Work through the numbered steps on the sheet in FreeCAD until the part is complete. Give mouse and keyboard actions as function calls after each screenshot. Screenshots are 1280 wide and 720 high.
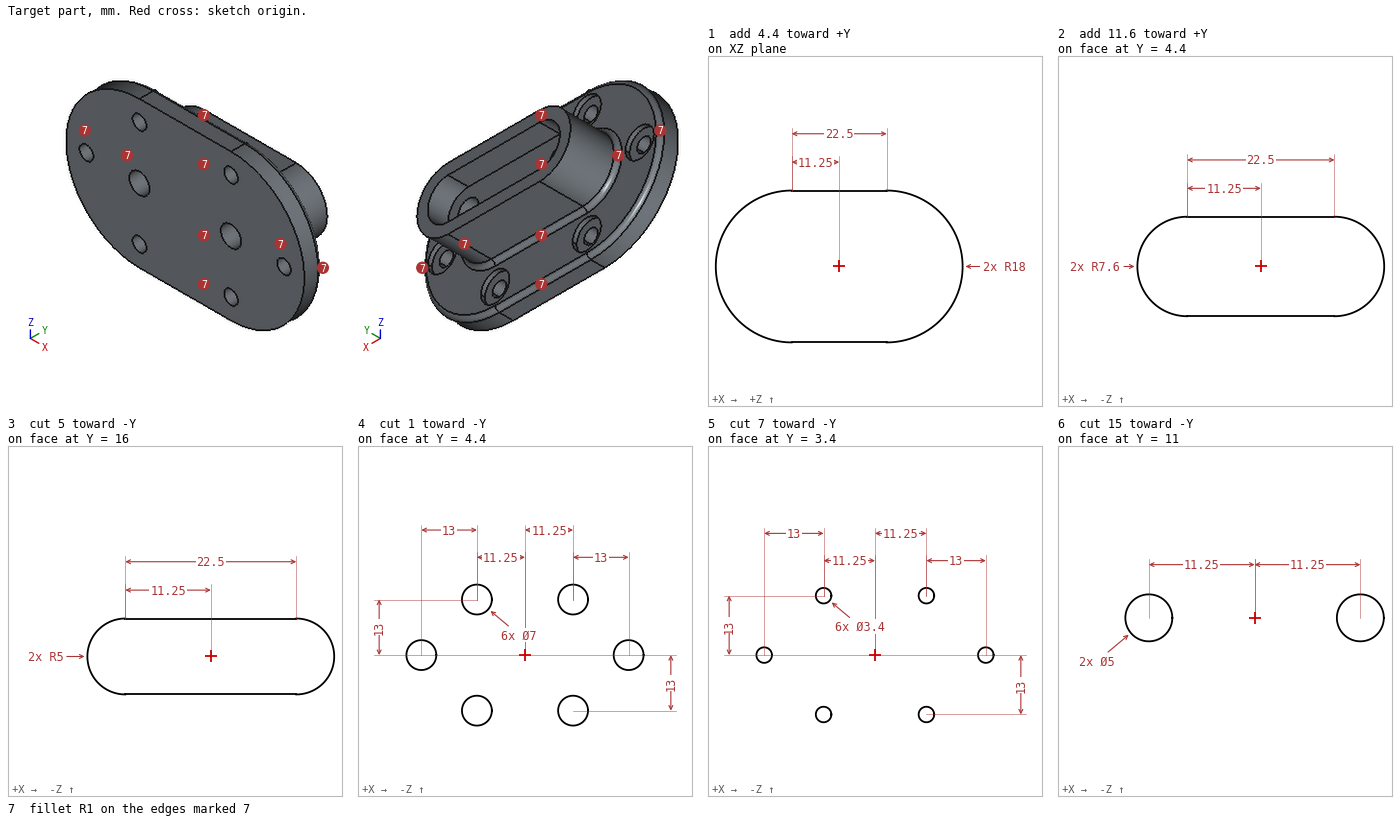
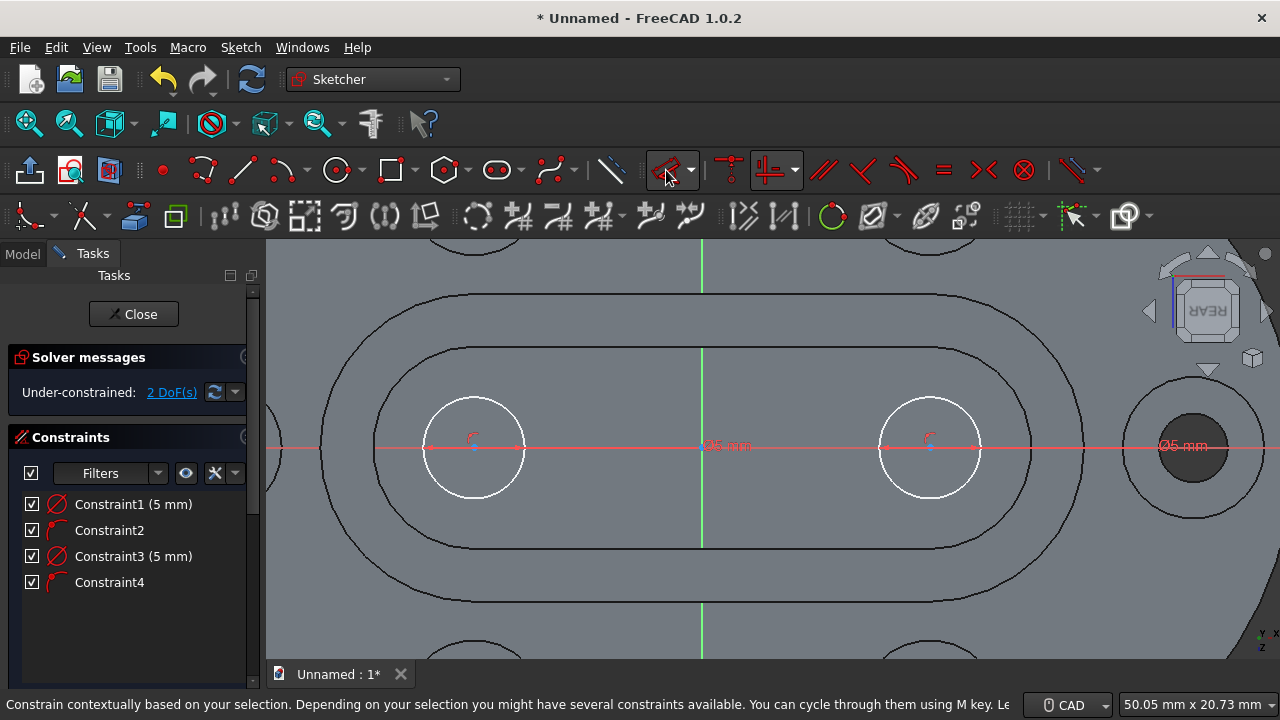
click(474, 448)
click(588, 482)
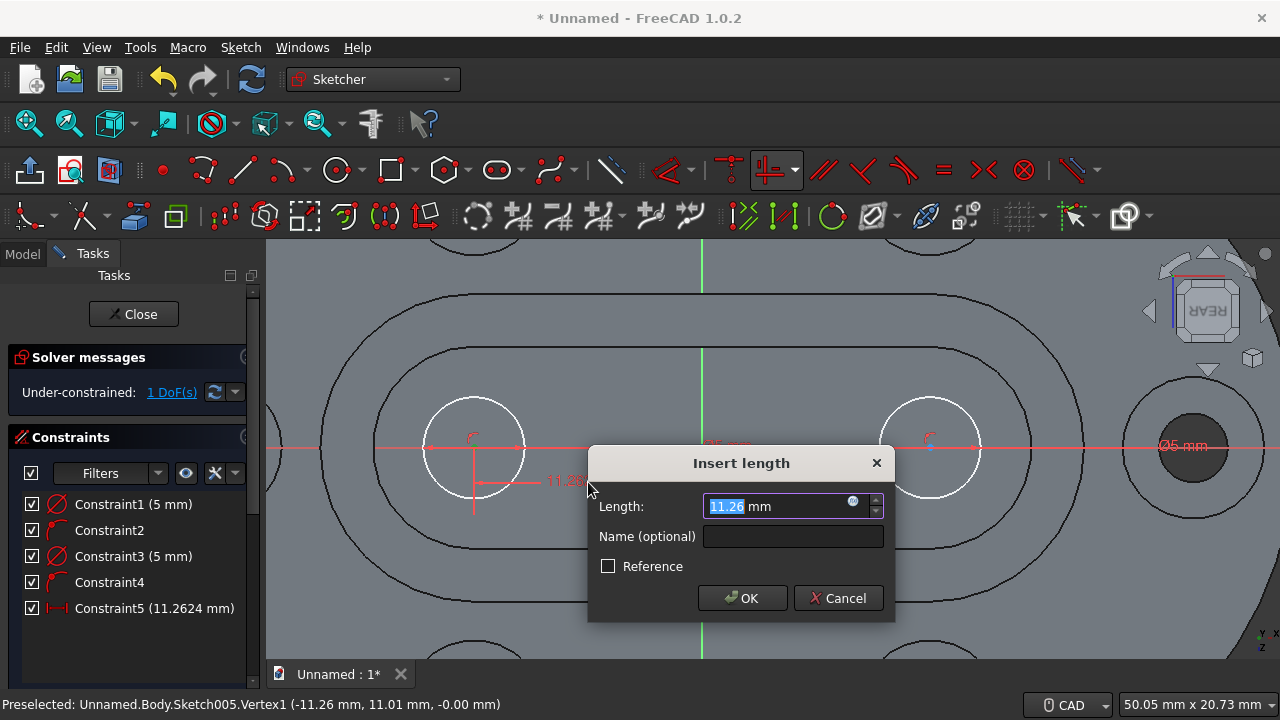
text(11.25)
key(Return)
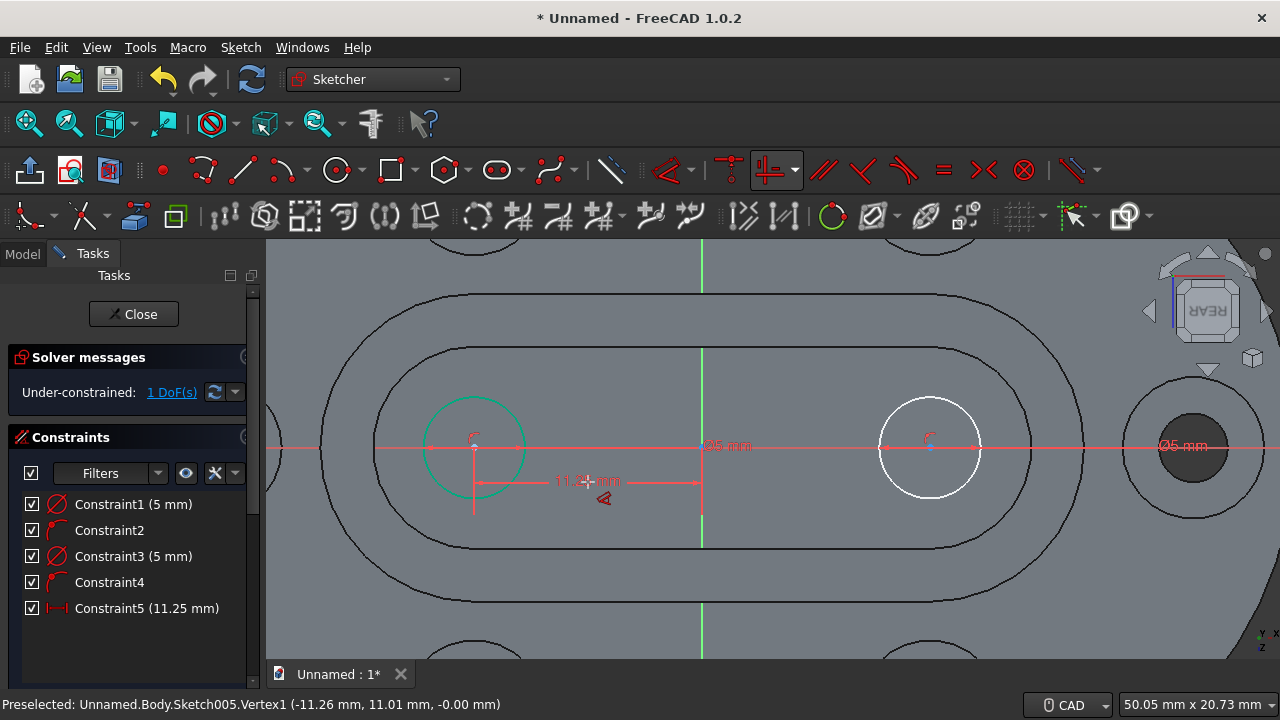
click(930, 448)
click(816, 482)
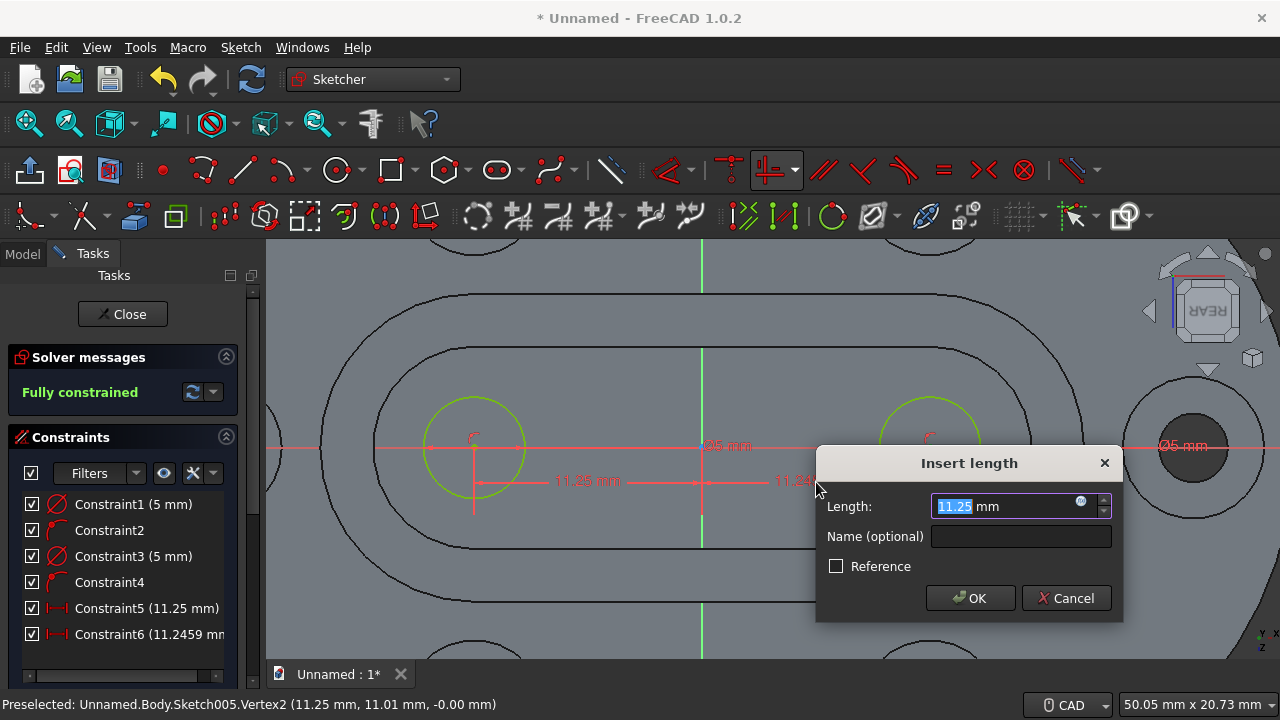
text(11.25)
key(Return)
key(Escape)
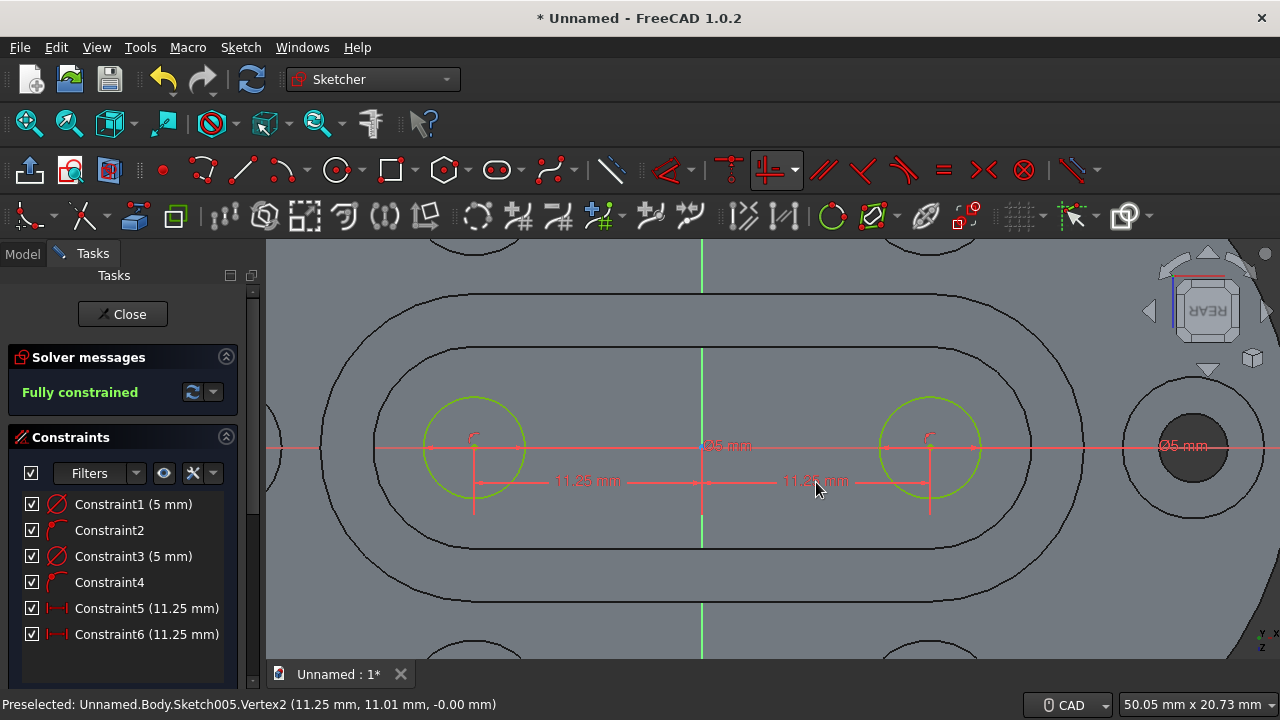
click(123, 314)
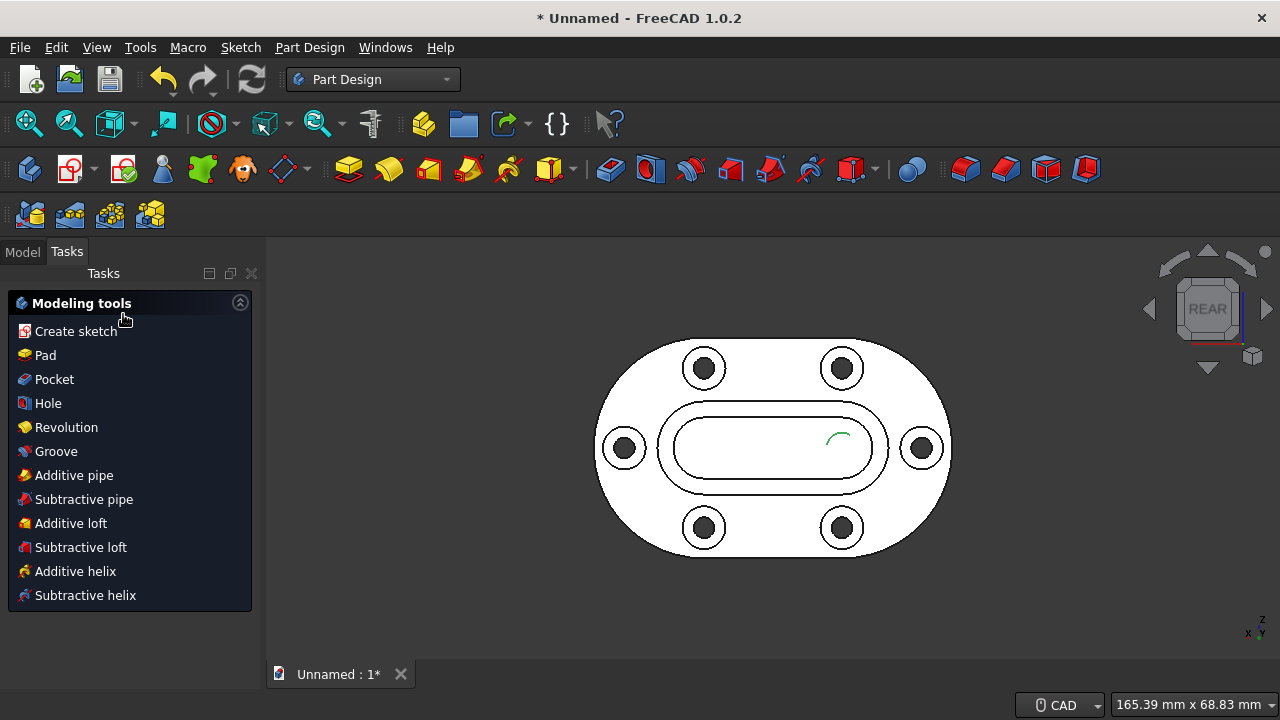
click(612, 170)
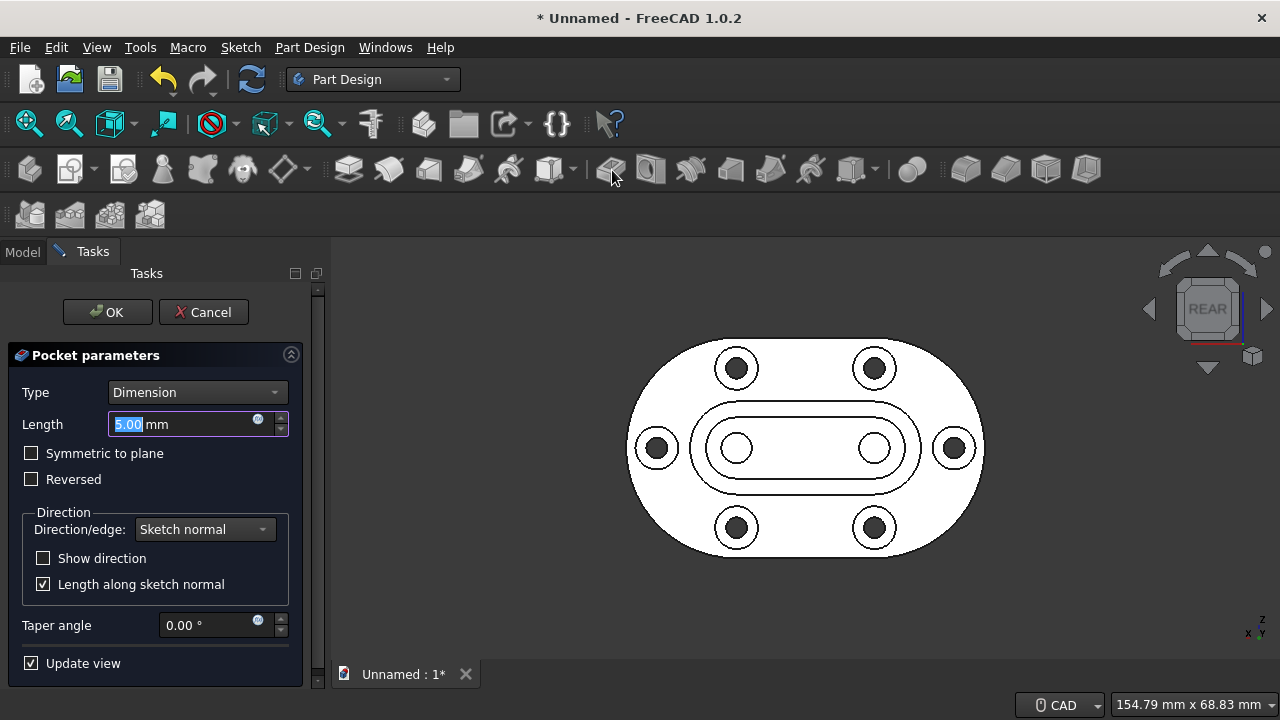
text(15)
key(Tab)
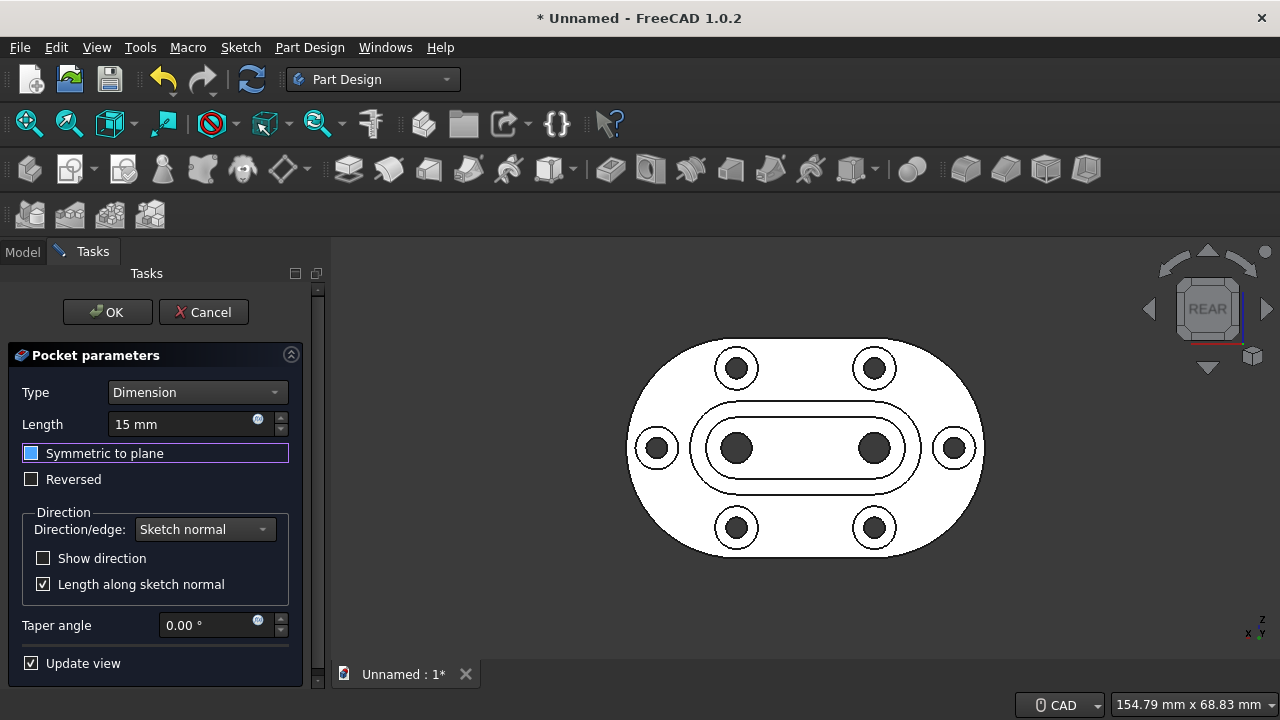
click(108, 312)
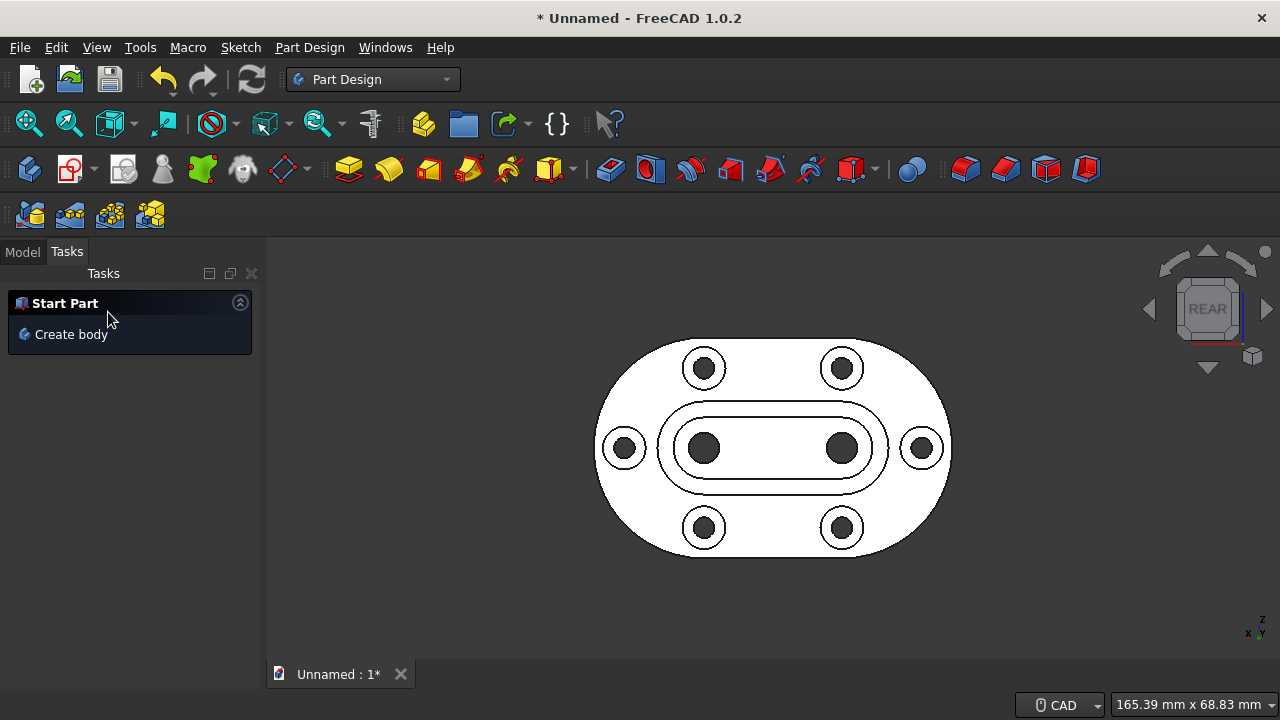
click(952, 447)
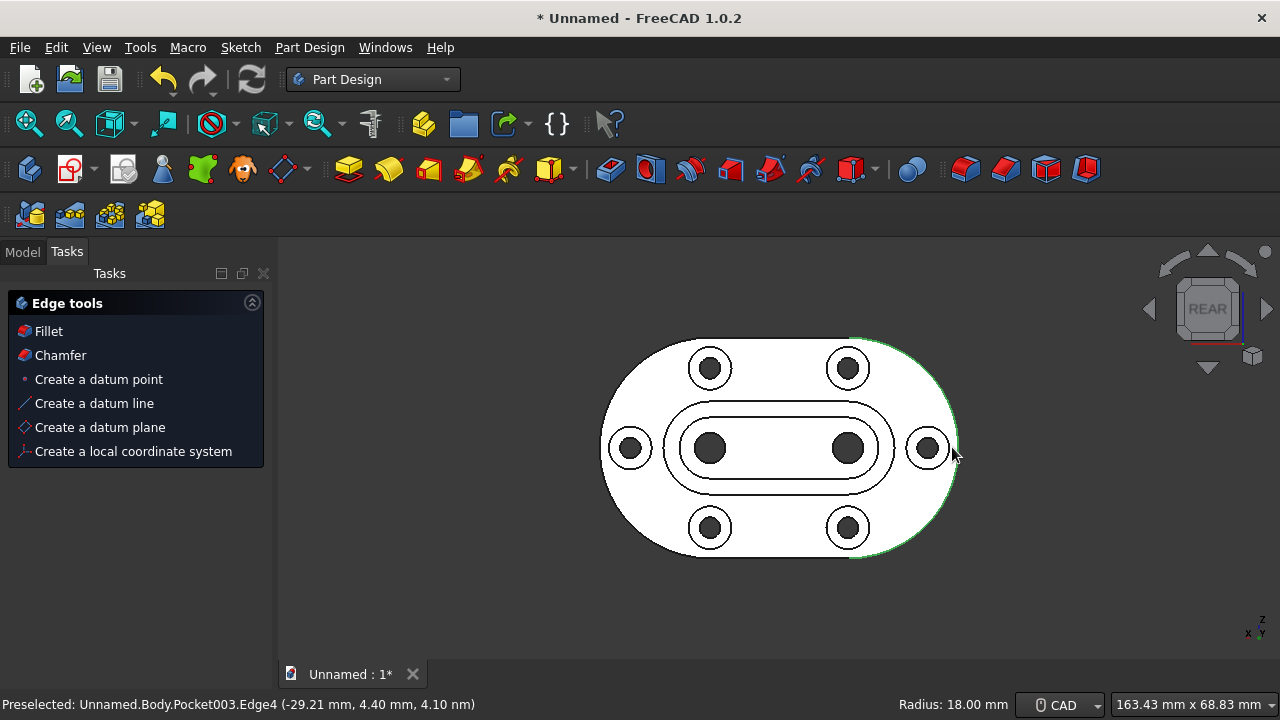
click(621, 512, ctrl)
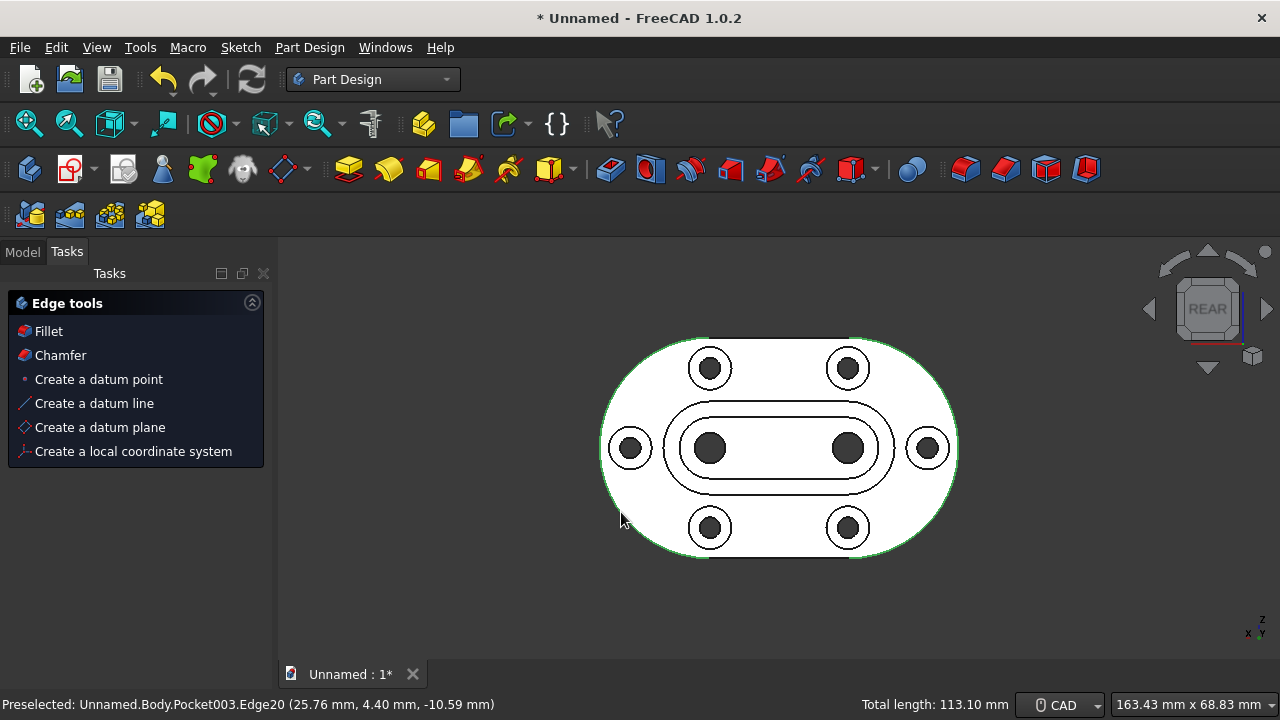
click(779, 557, ctrl)